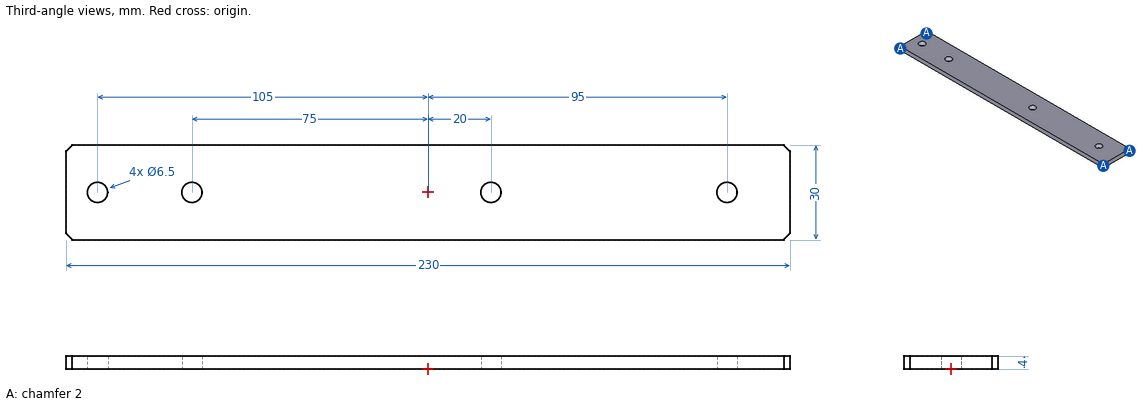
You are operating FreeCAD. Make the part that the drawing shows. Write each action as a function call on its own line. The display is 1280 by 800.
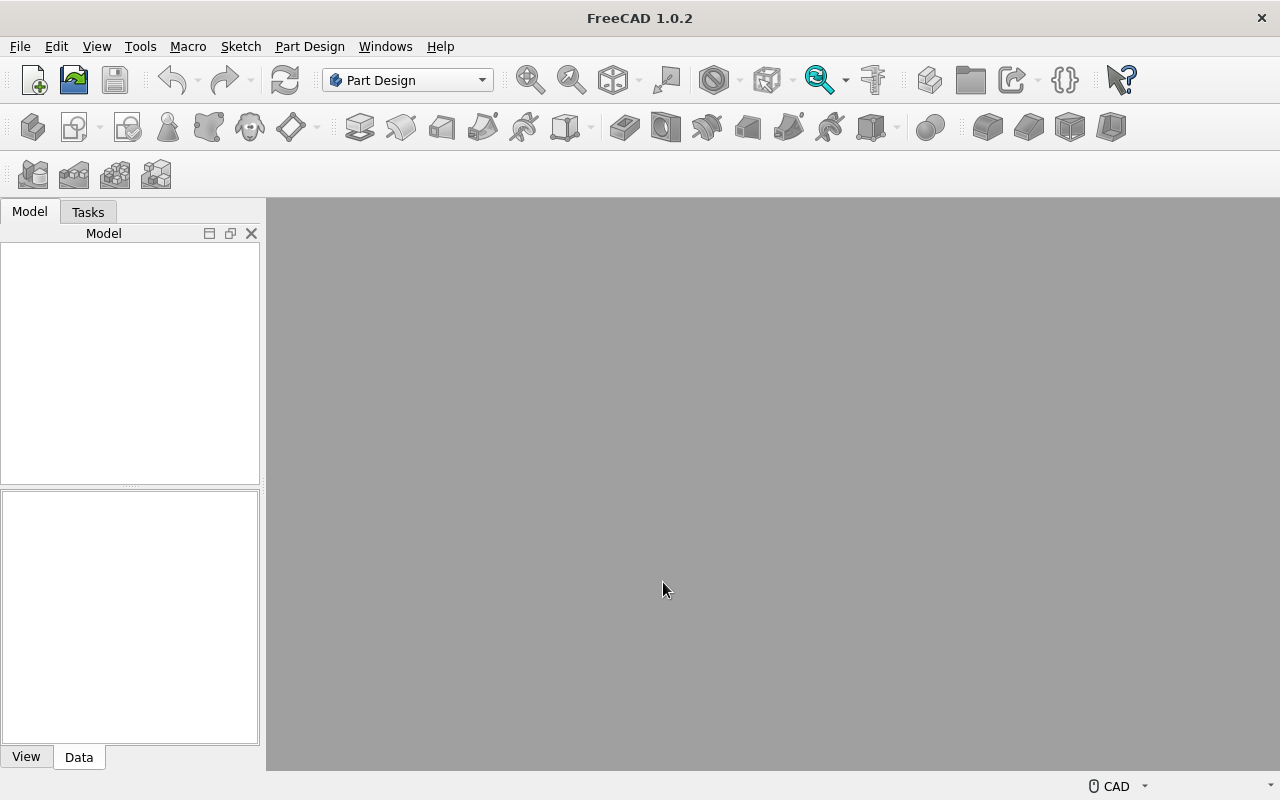
click(33, 80)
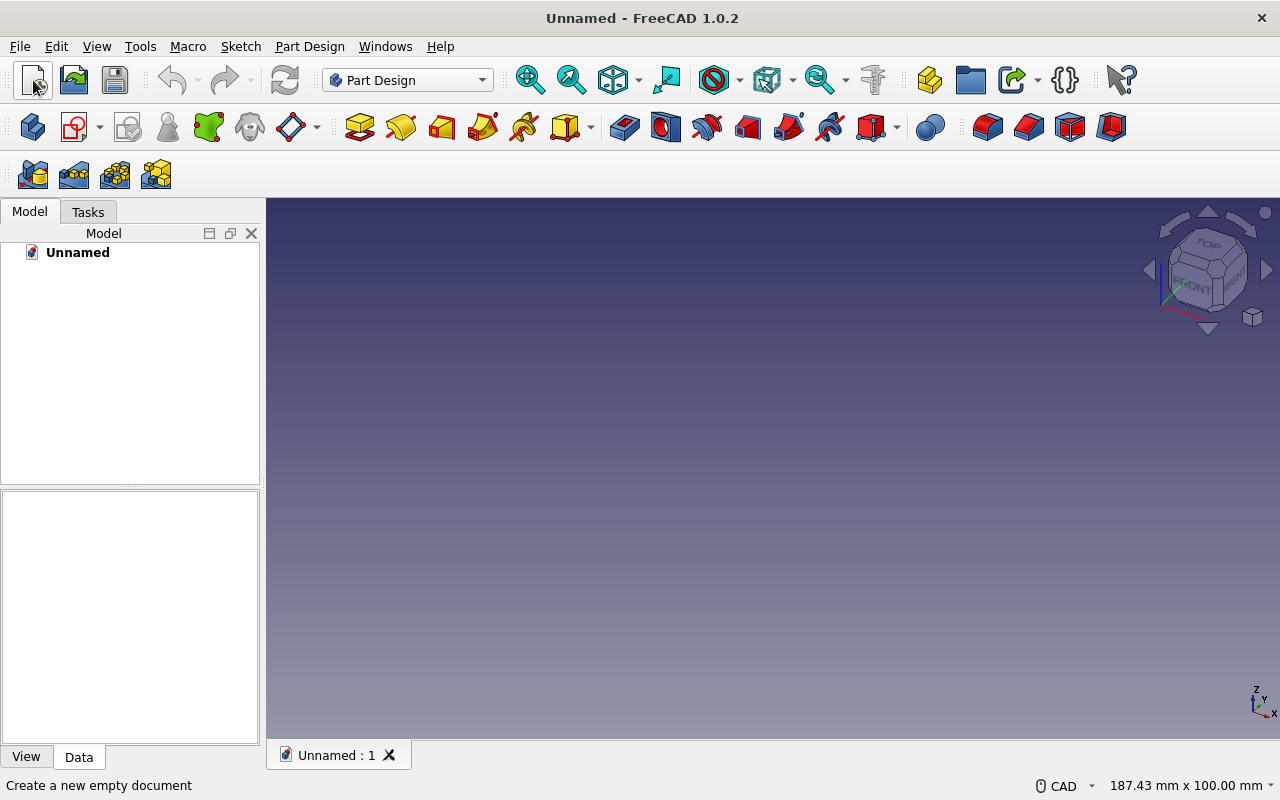
click(74, 128)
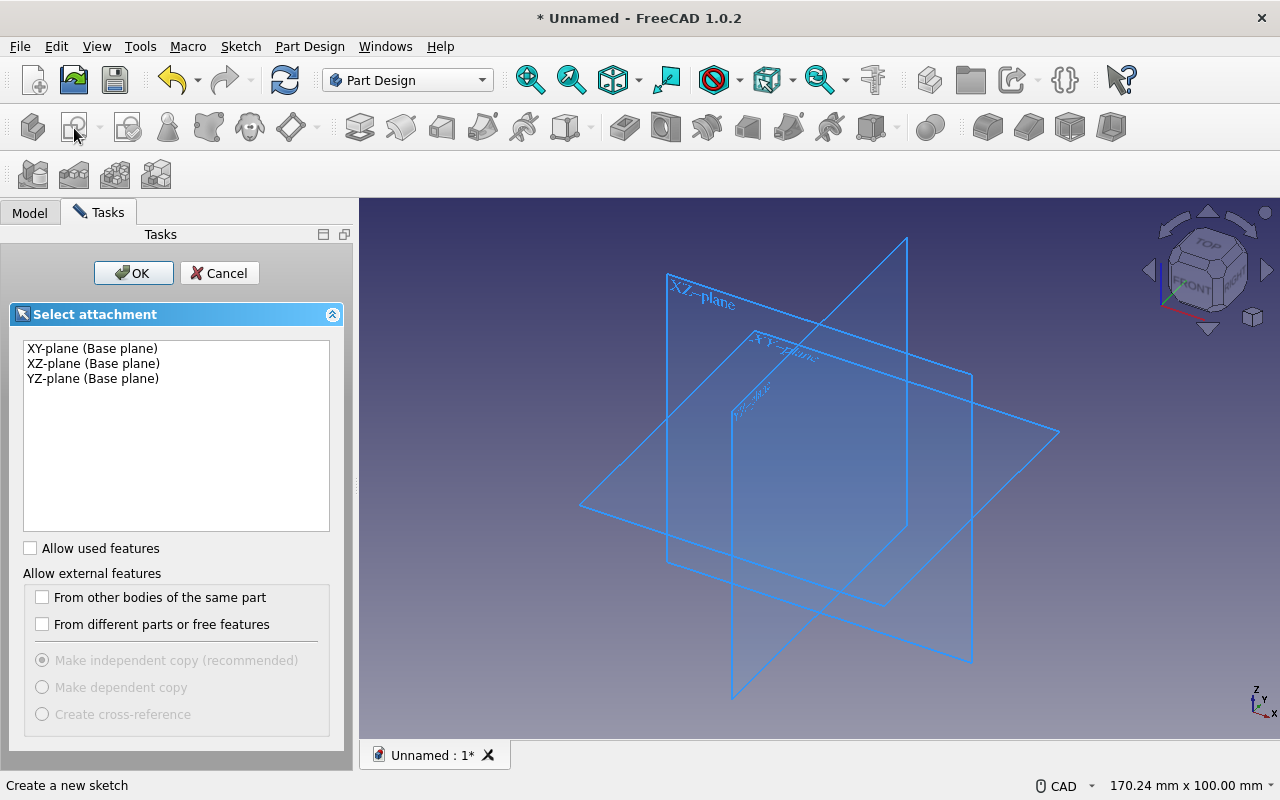
click(84, 348)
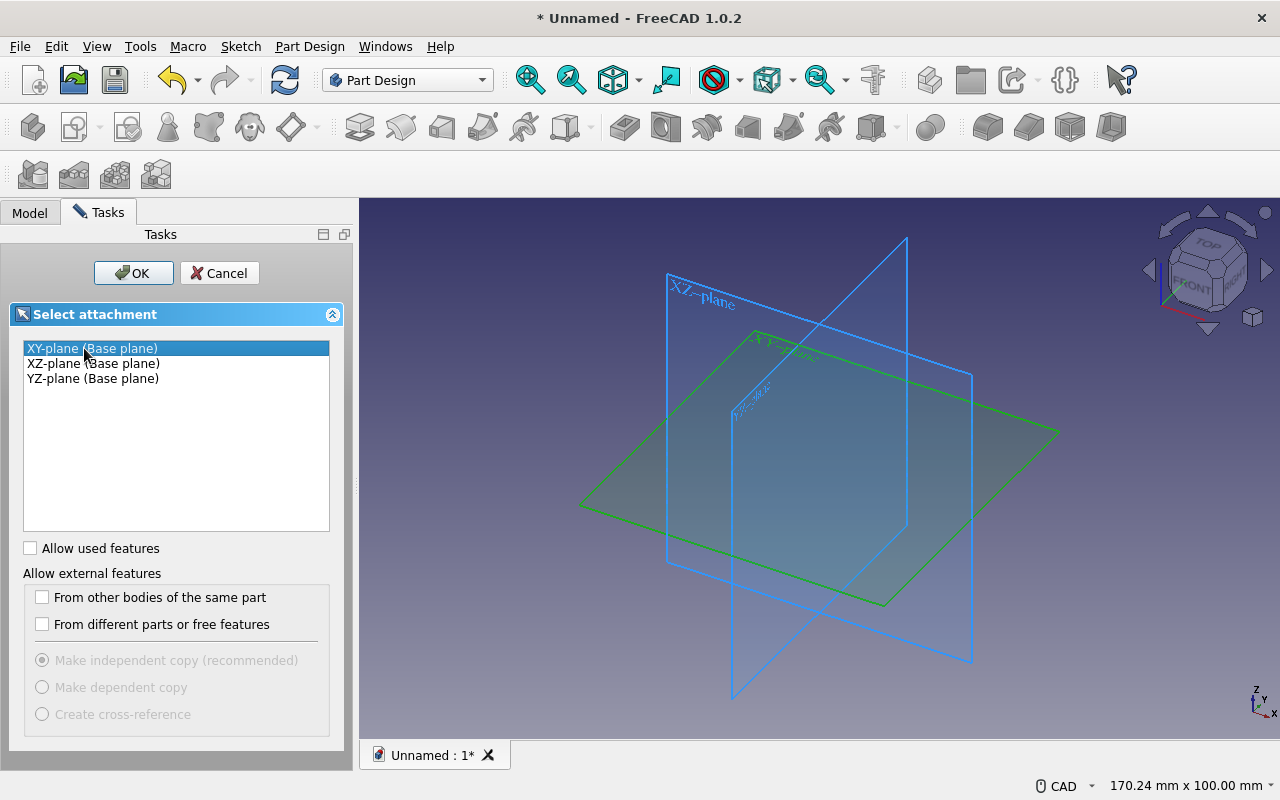
click(134, 273)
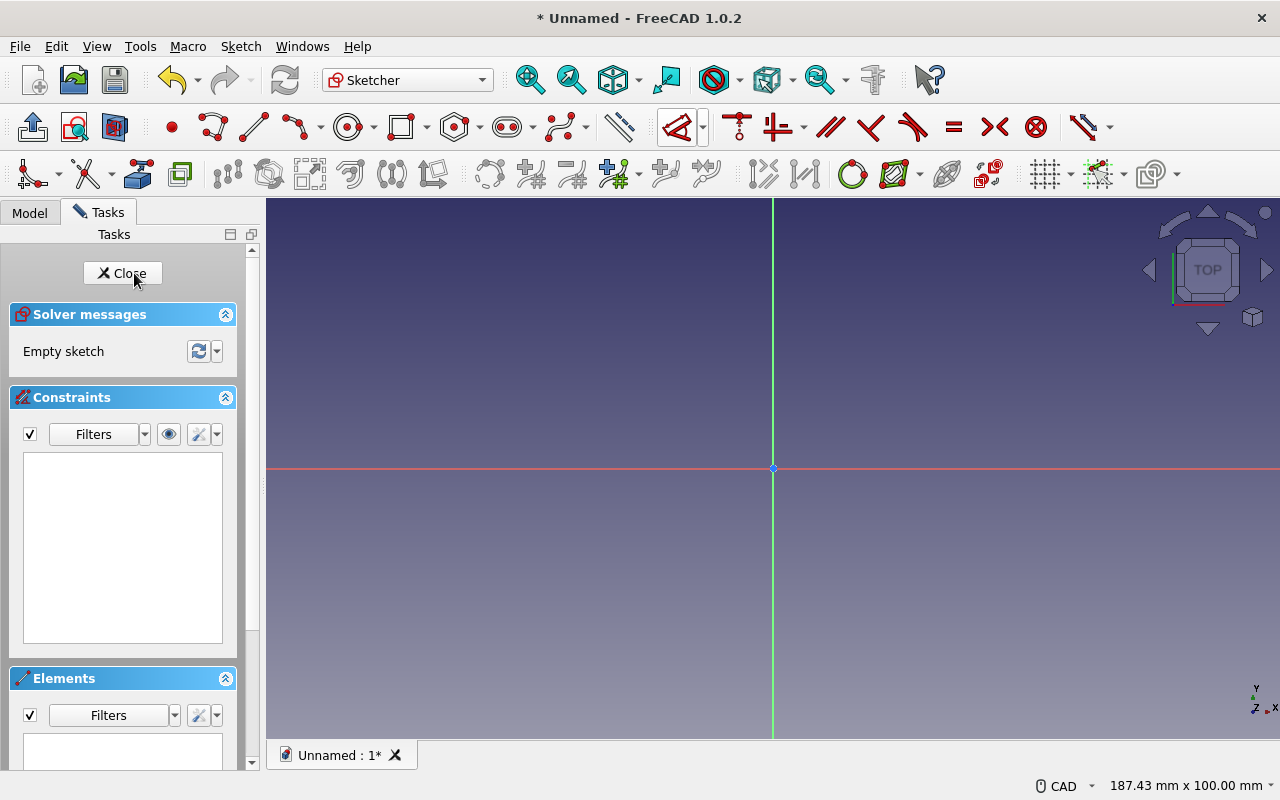
scroll(649, 469, down, 4)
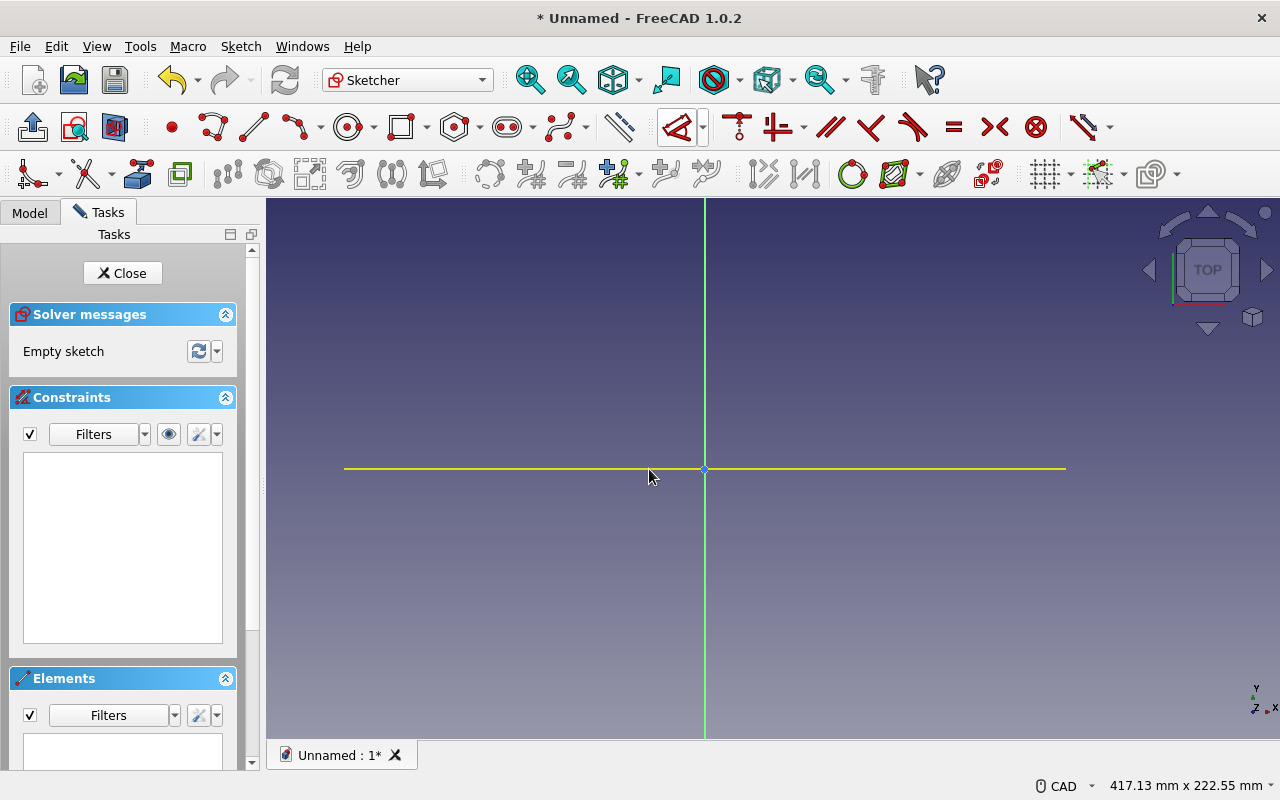
key(g)
key(v)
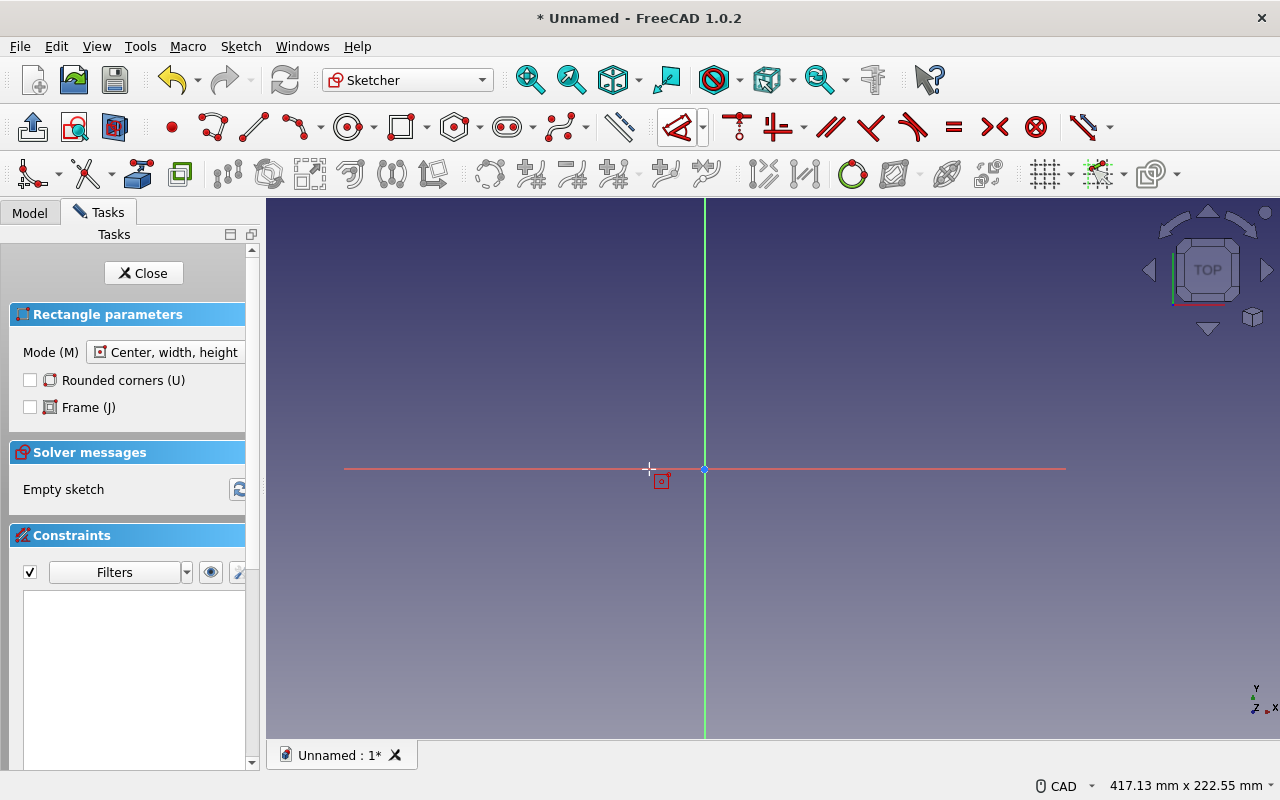
click(705, 469)
move(984, 433)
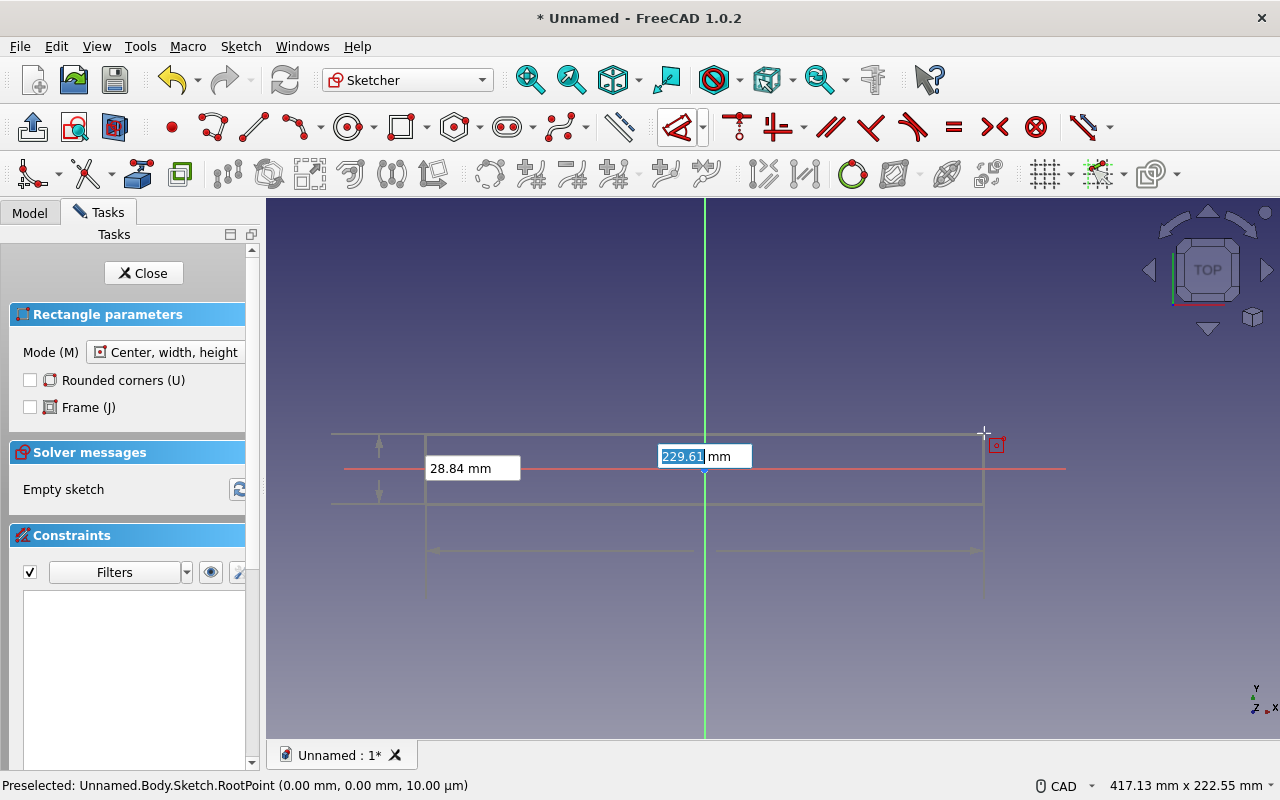
text(230)
key(Tab)
text(30)
key(Return)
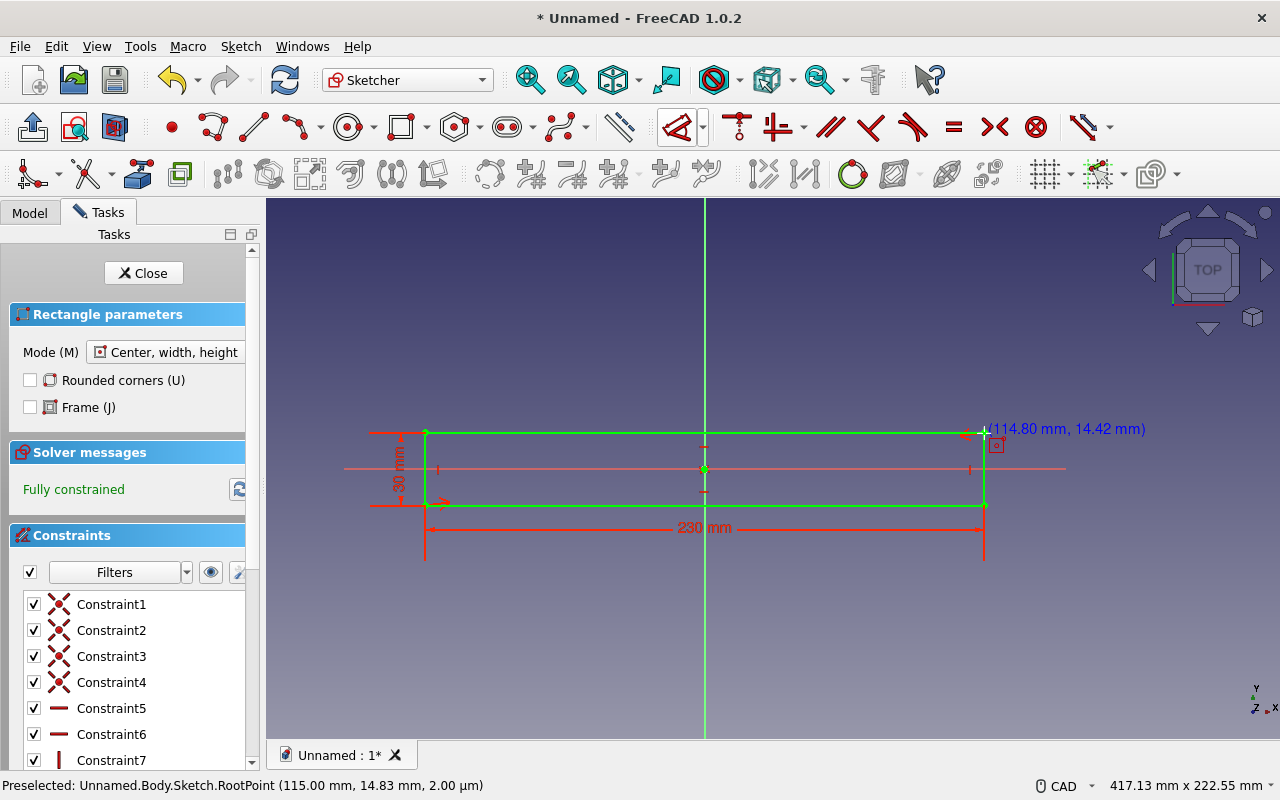
click(348, 128)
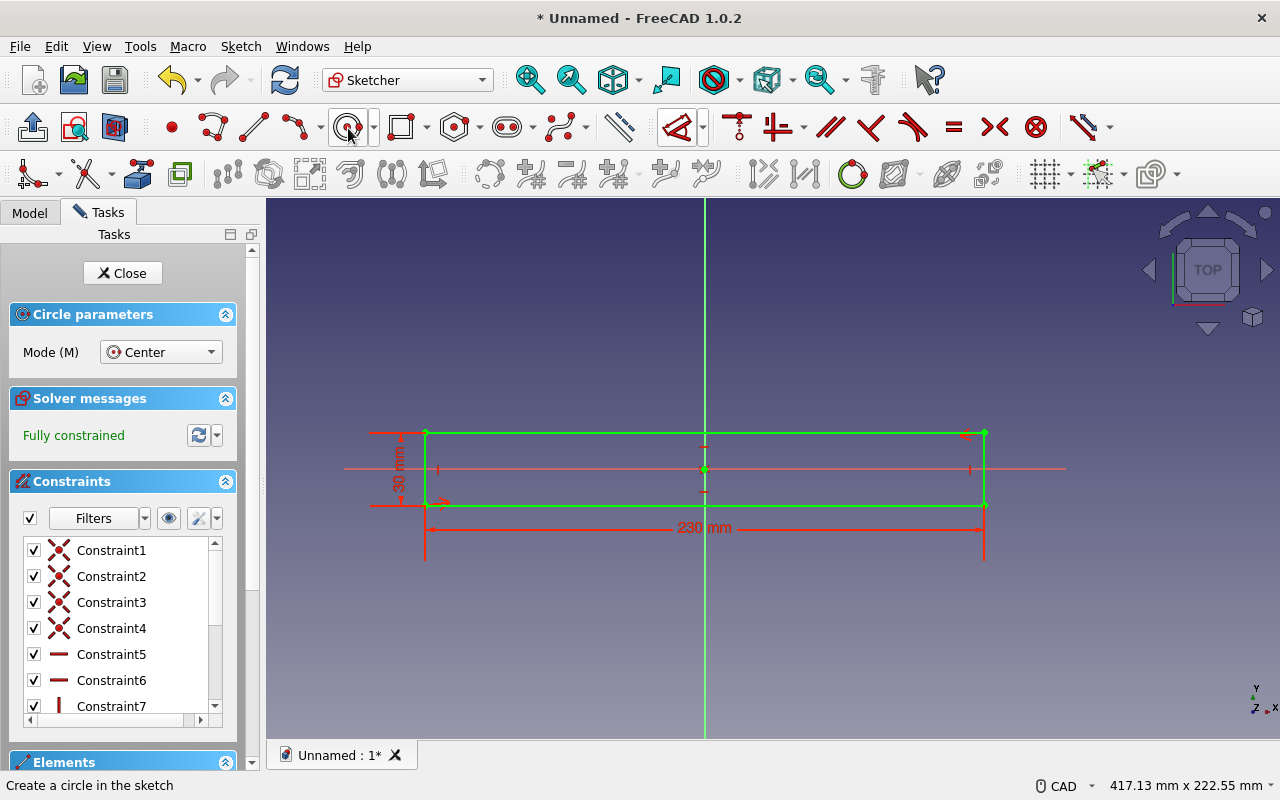
scroll(450, 469, up, 6)